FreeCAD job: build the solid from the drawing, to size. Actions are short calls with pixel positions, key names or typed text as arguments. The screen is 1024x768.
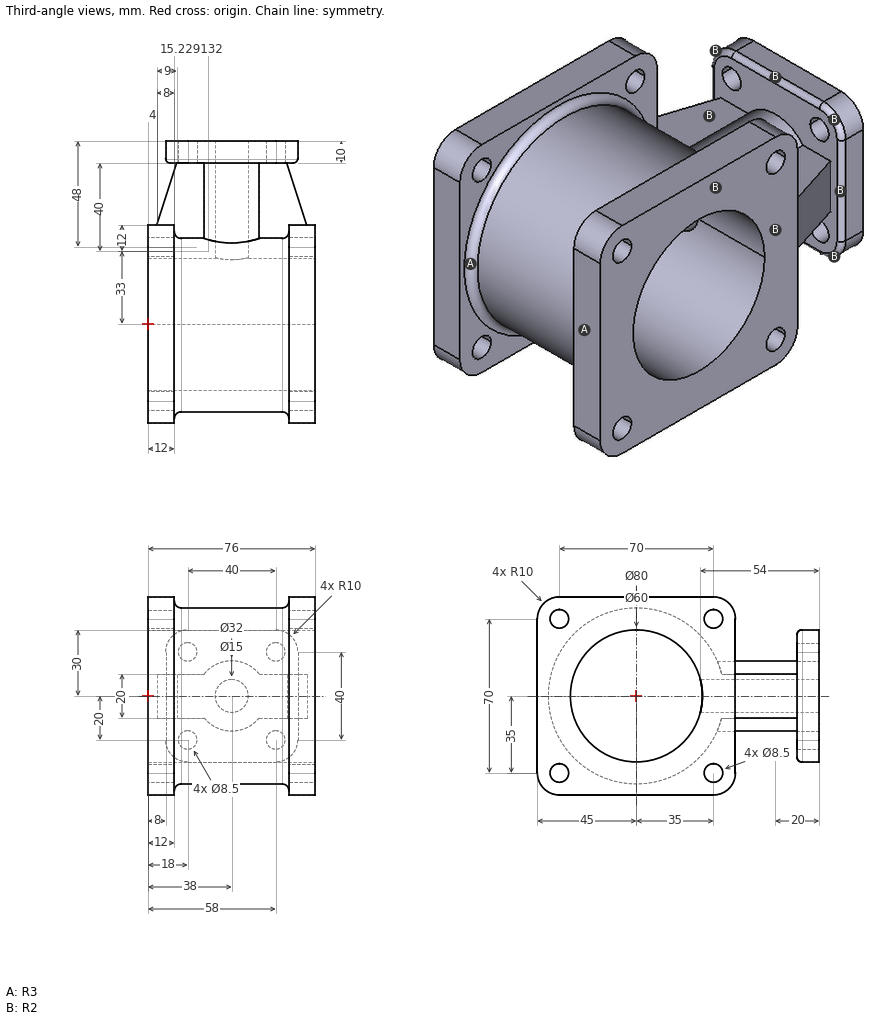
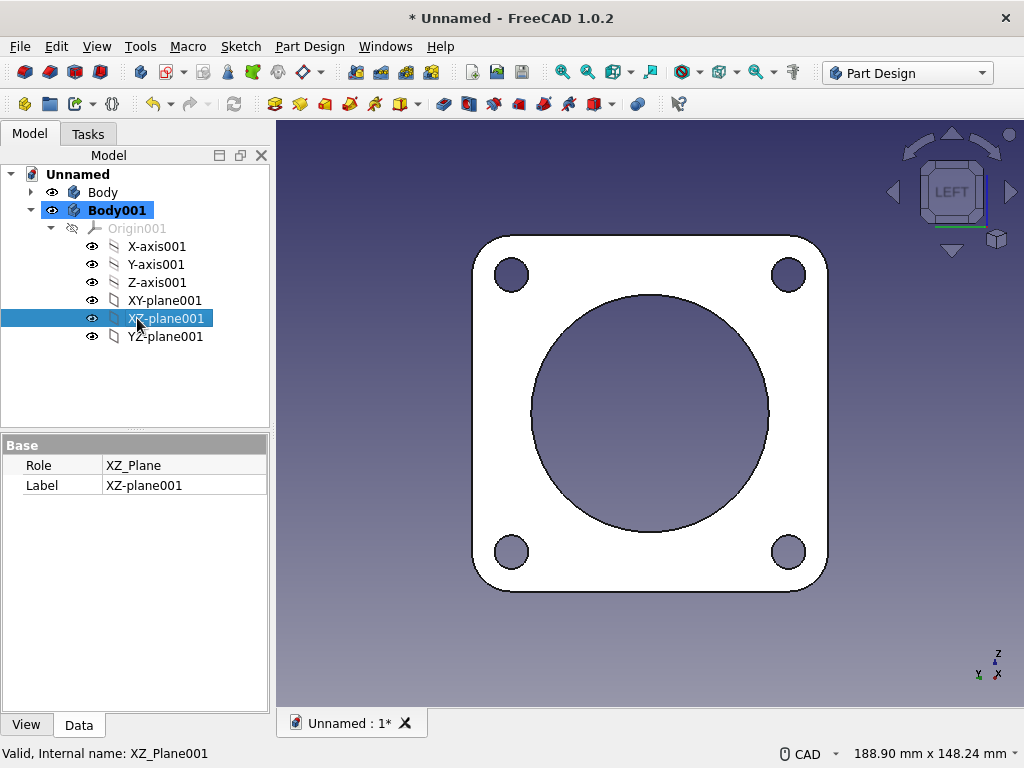
click(302, 72)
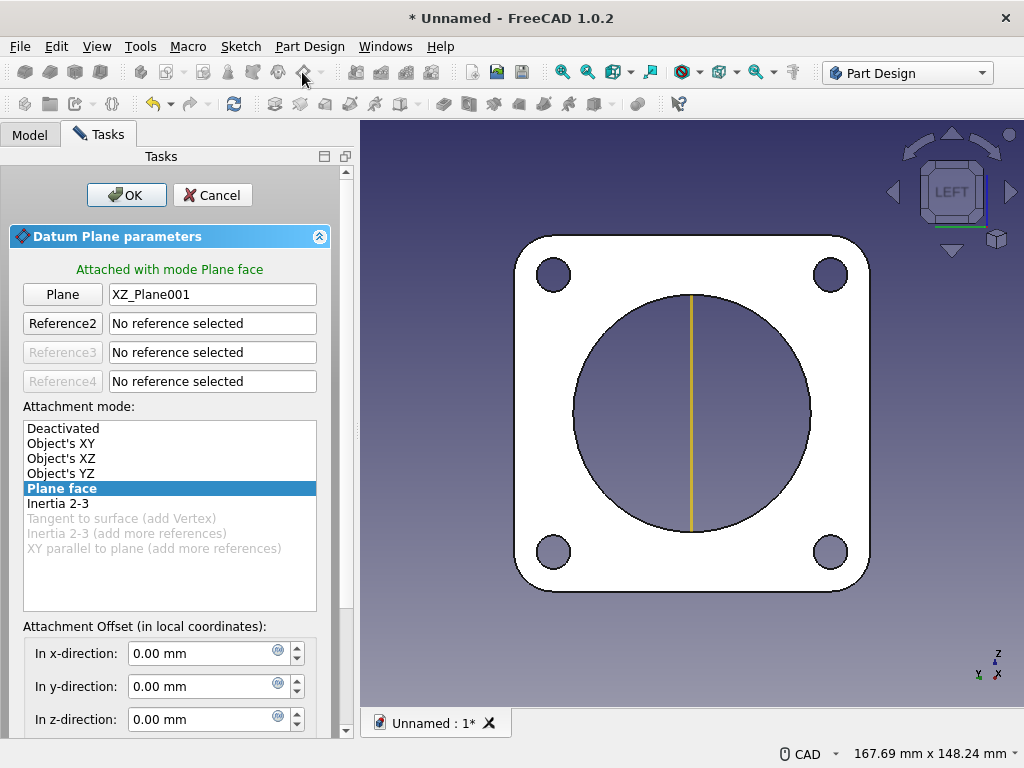
triple_click(210, 720)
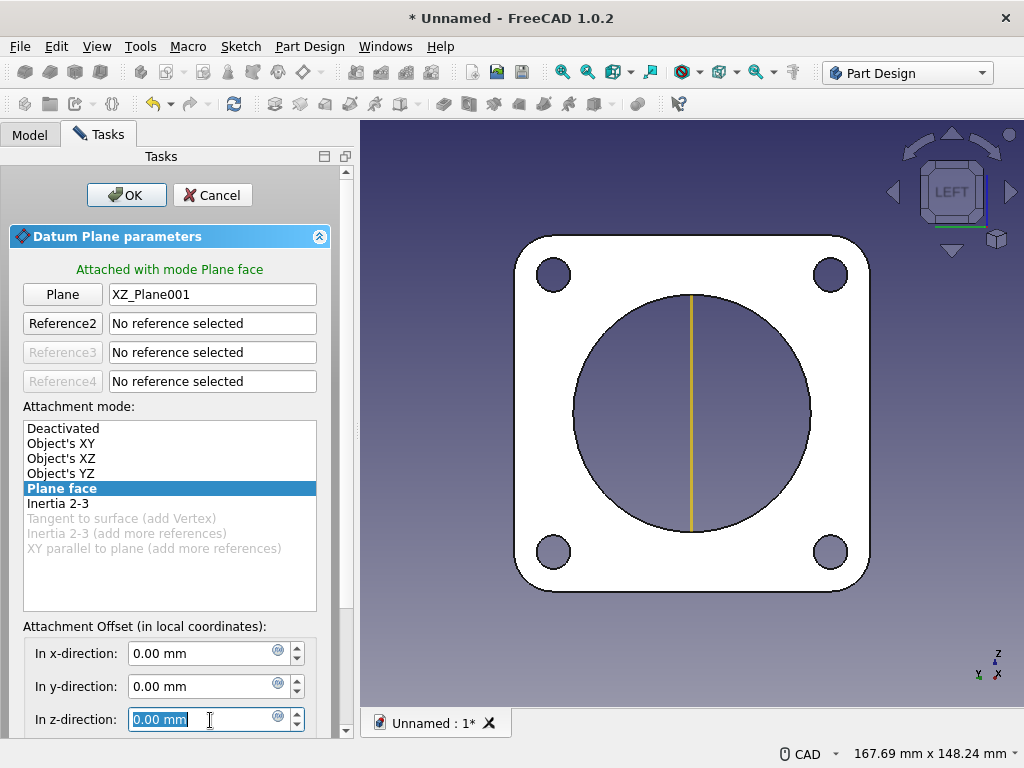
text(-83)
key(Tab)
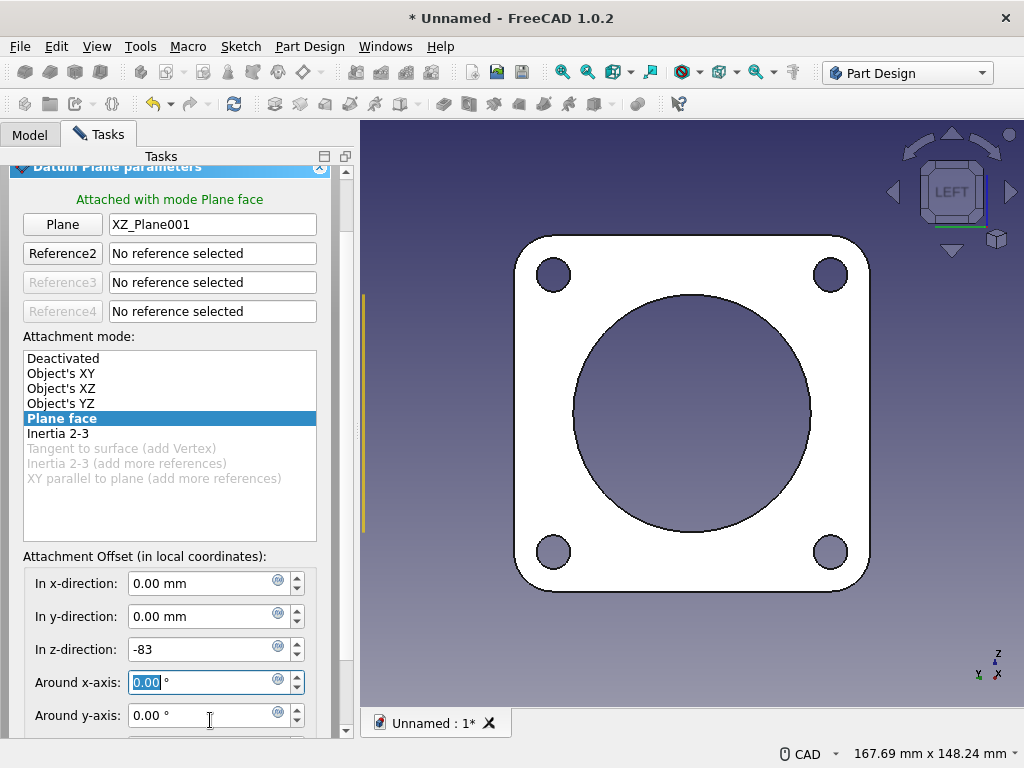
scroll(346, 452, up, 2)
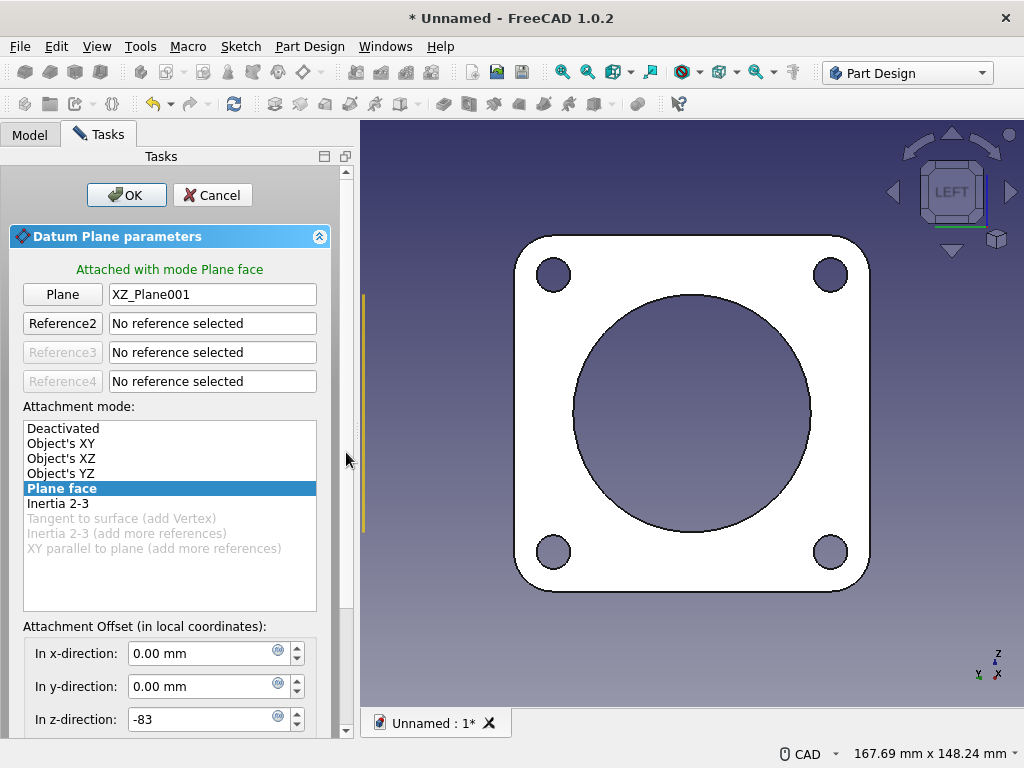
click(127, 195)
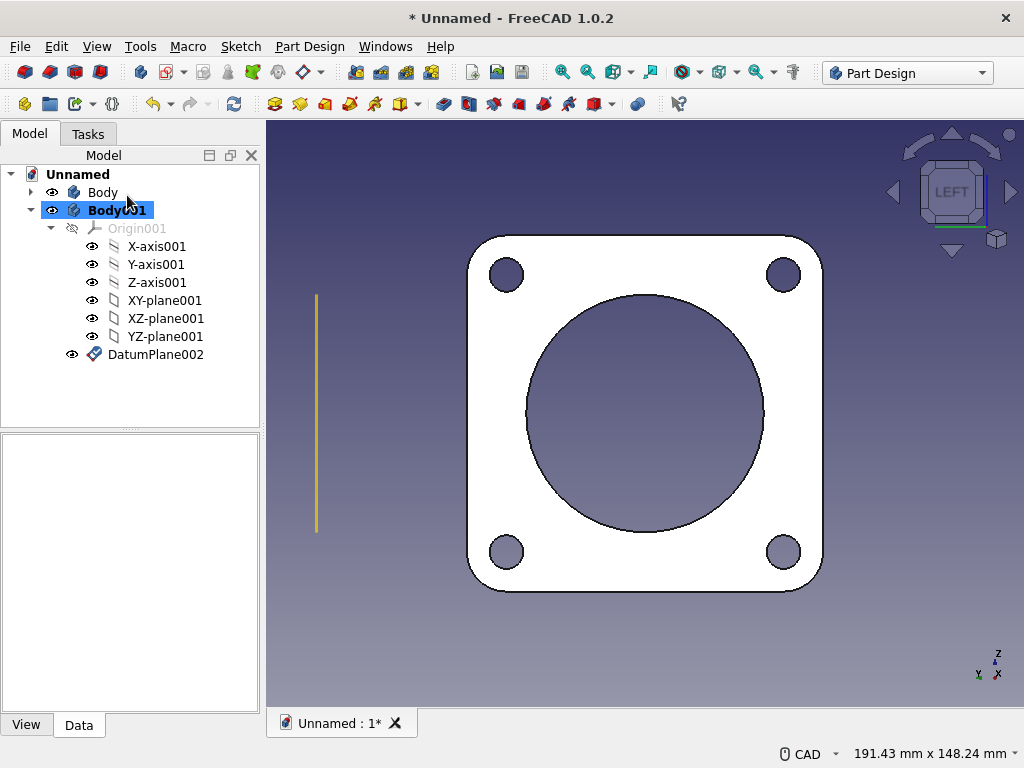
click(117, 354)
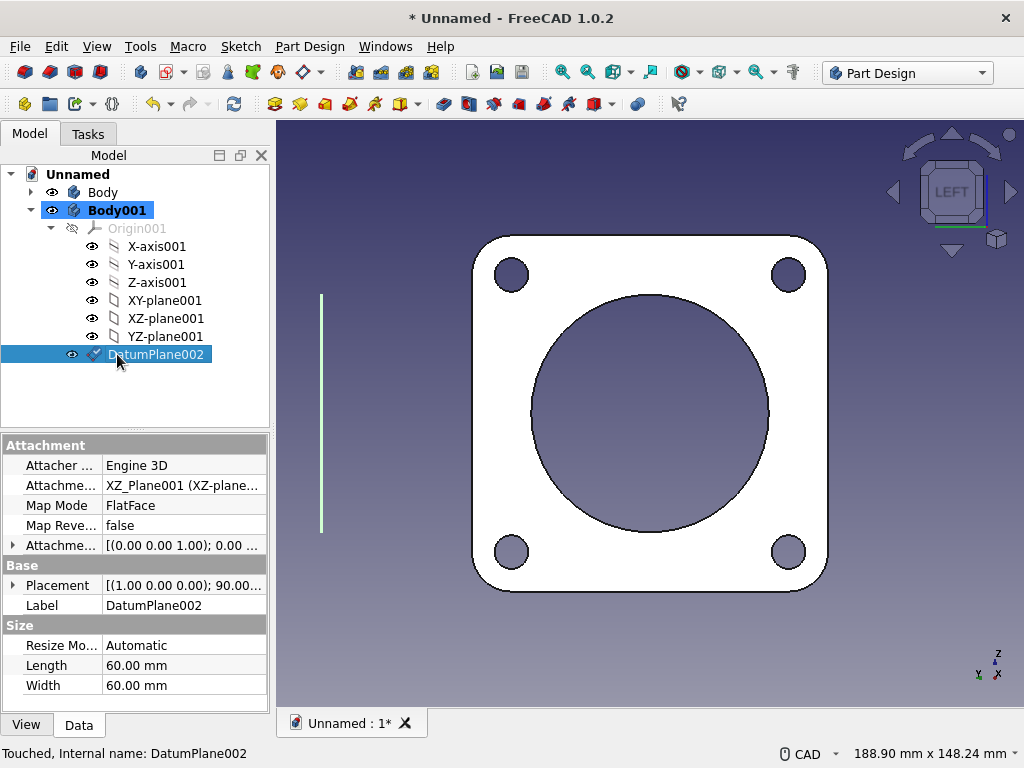
click(166, 72)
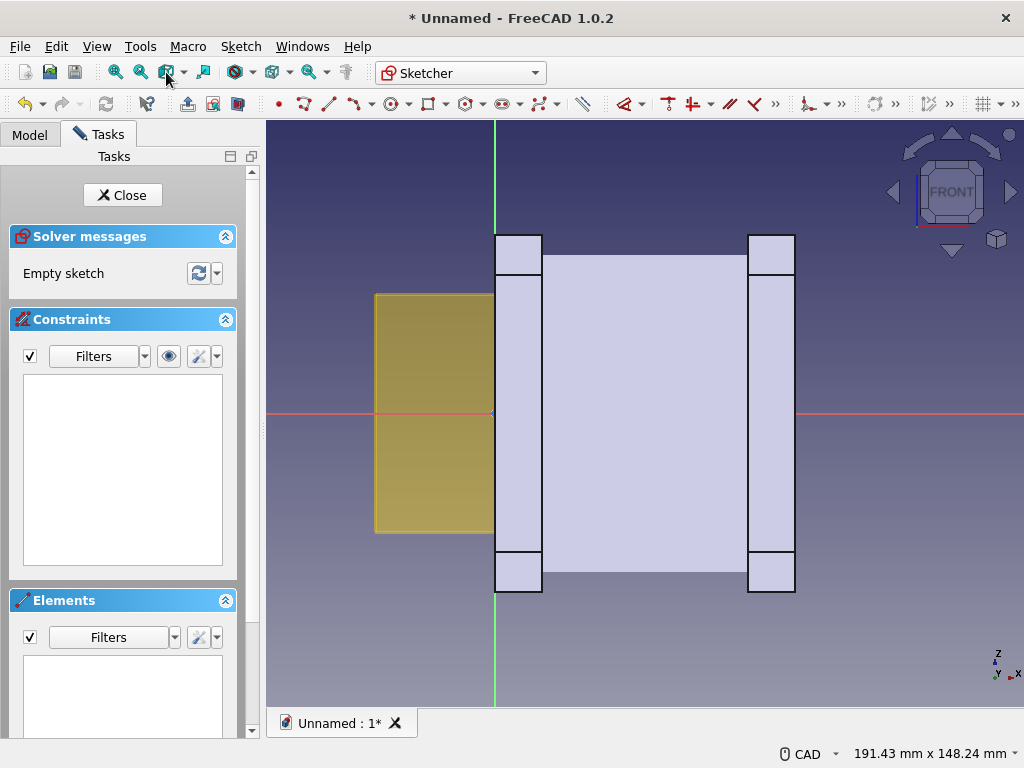
scroll(736, 414, up, 2)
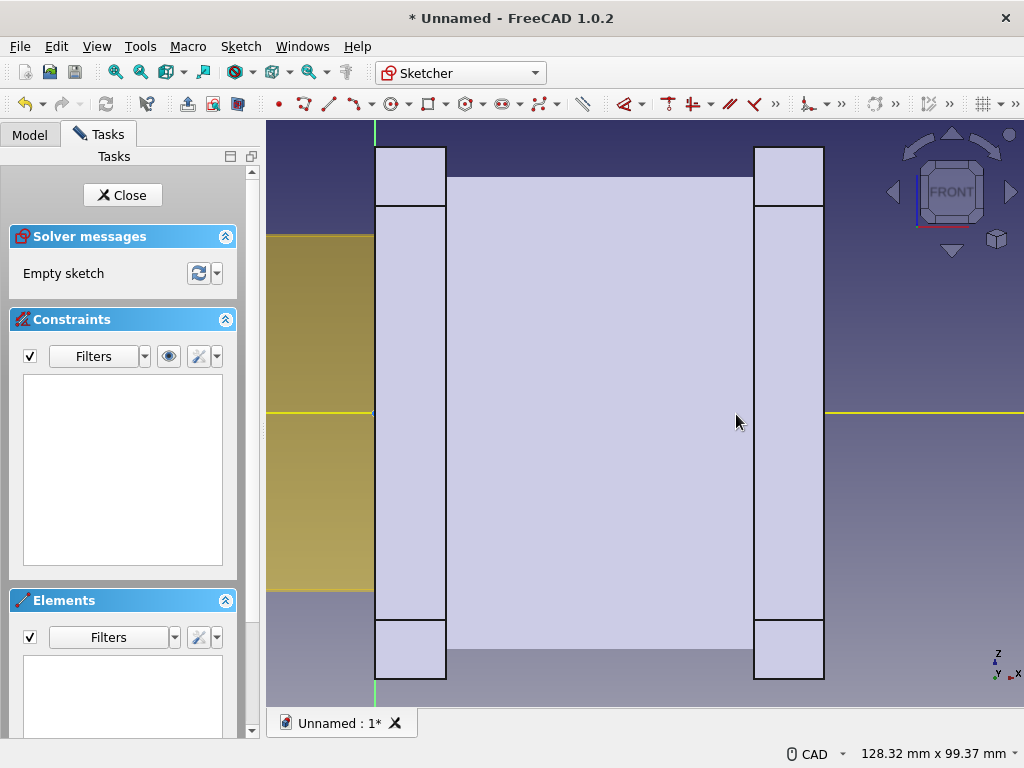
key(g)
key(l)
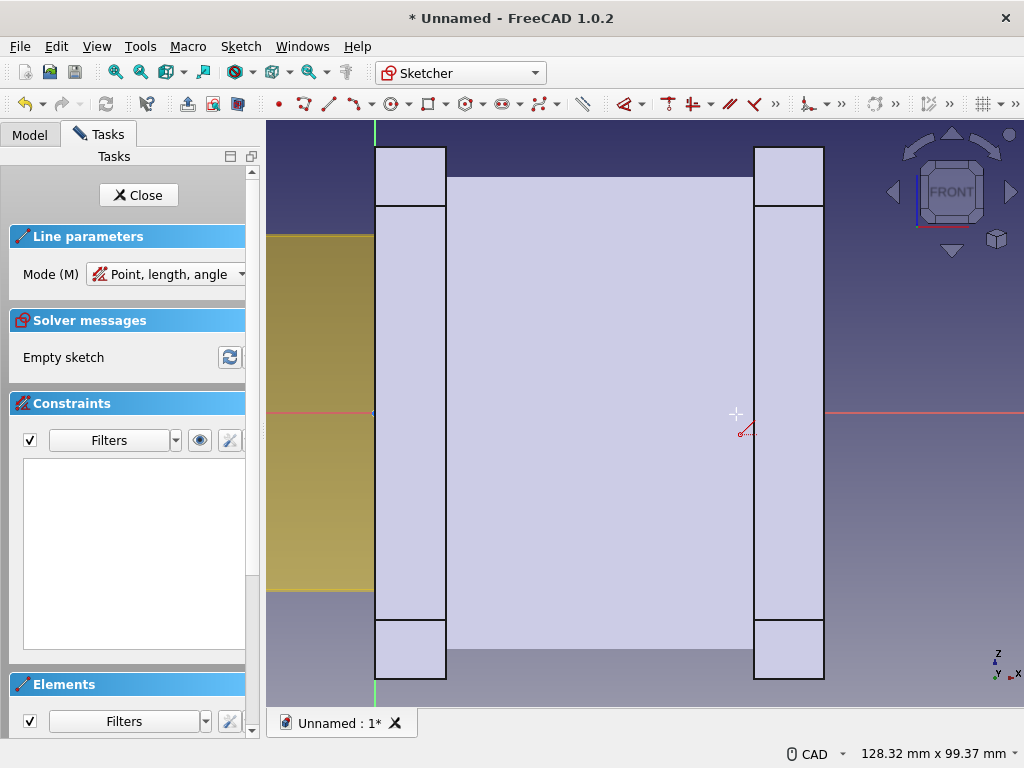
click(482, 236)
click(718, 236)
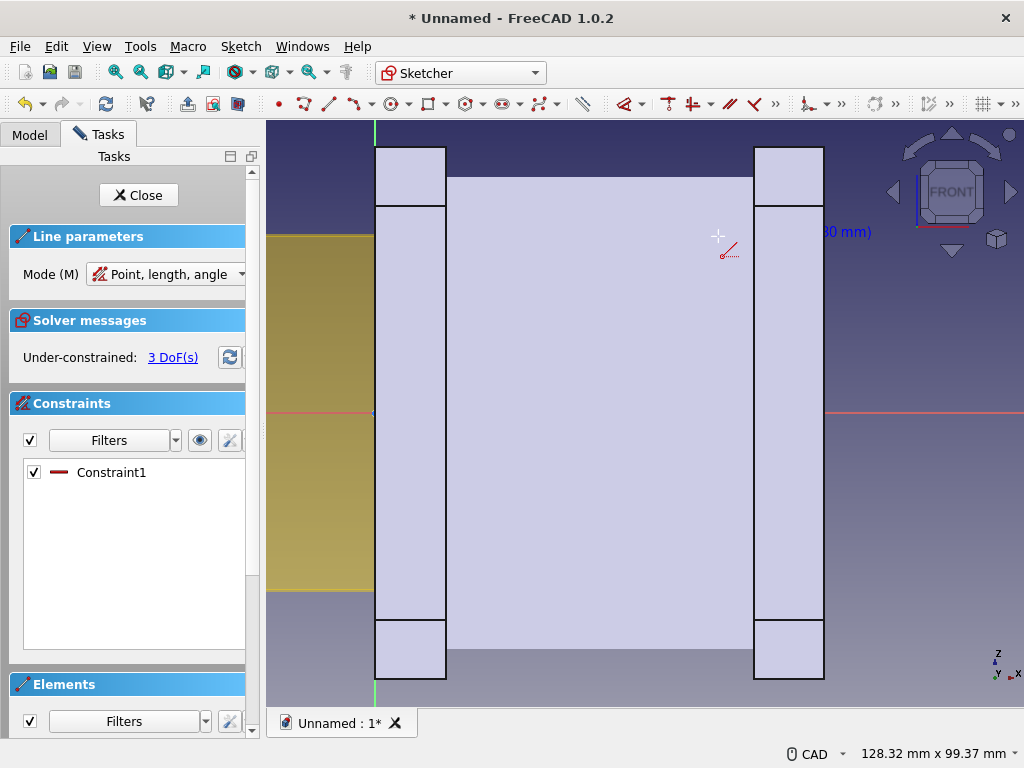
click(777, 295)
click(777, 531)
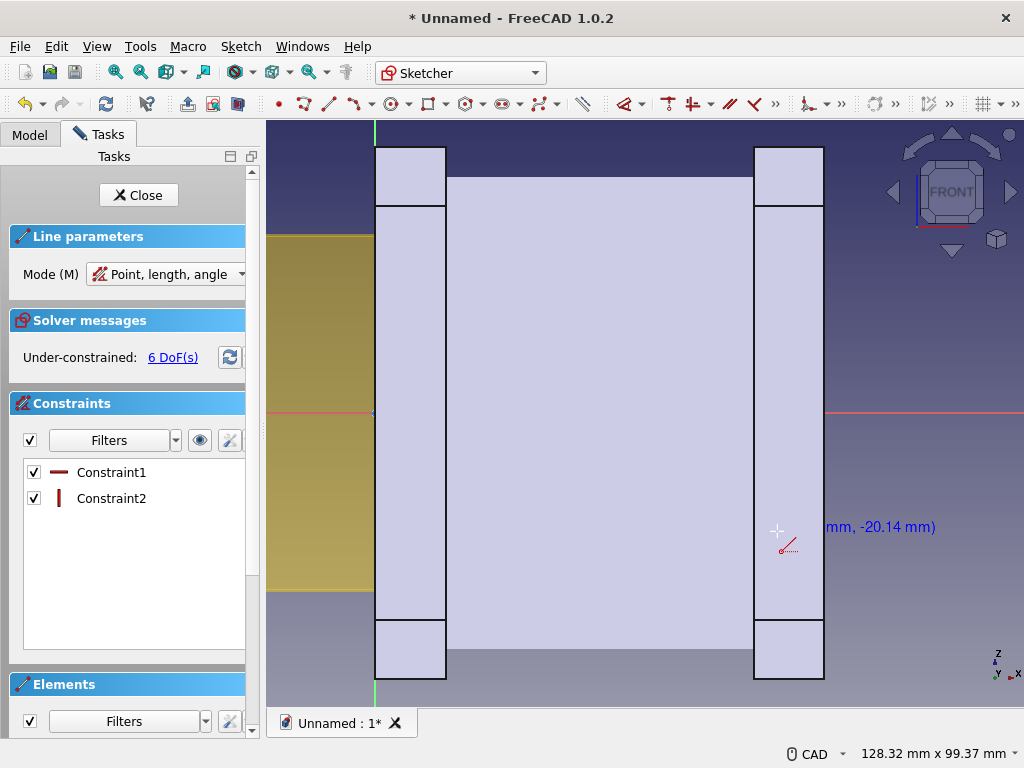
click(718, 590)
click(482, 590)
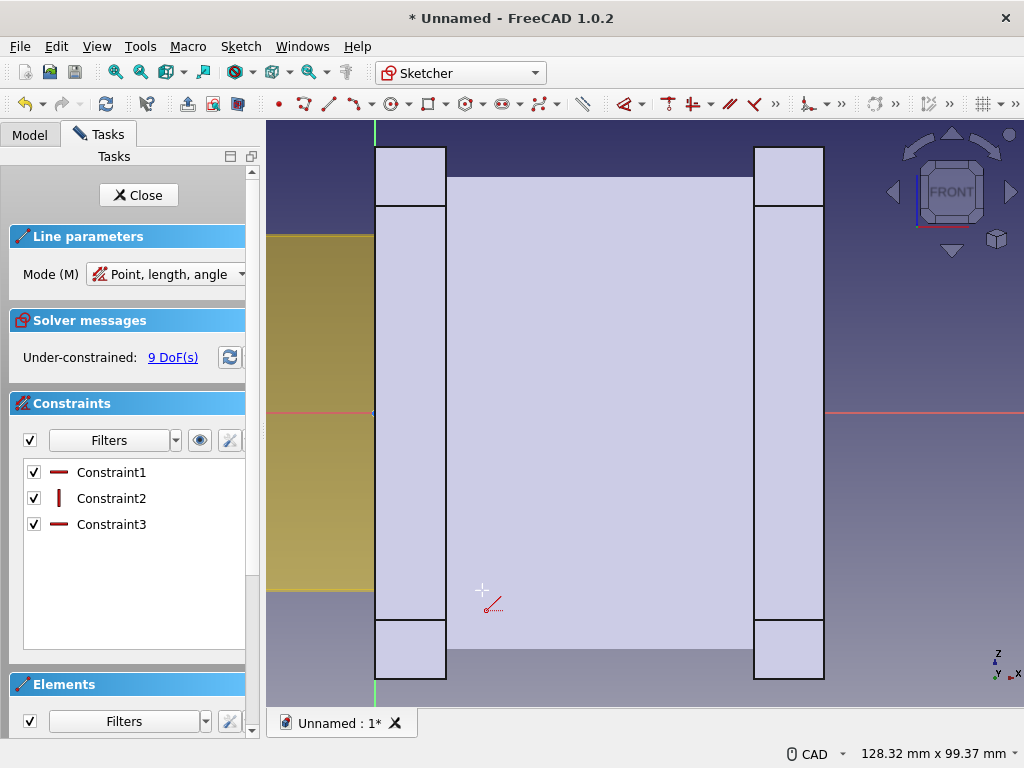
click(423, 531)
click(423, 295)